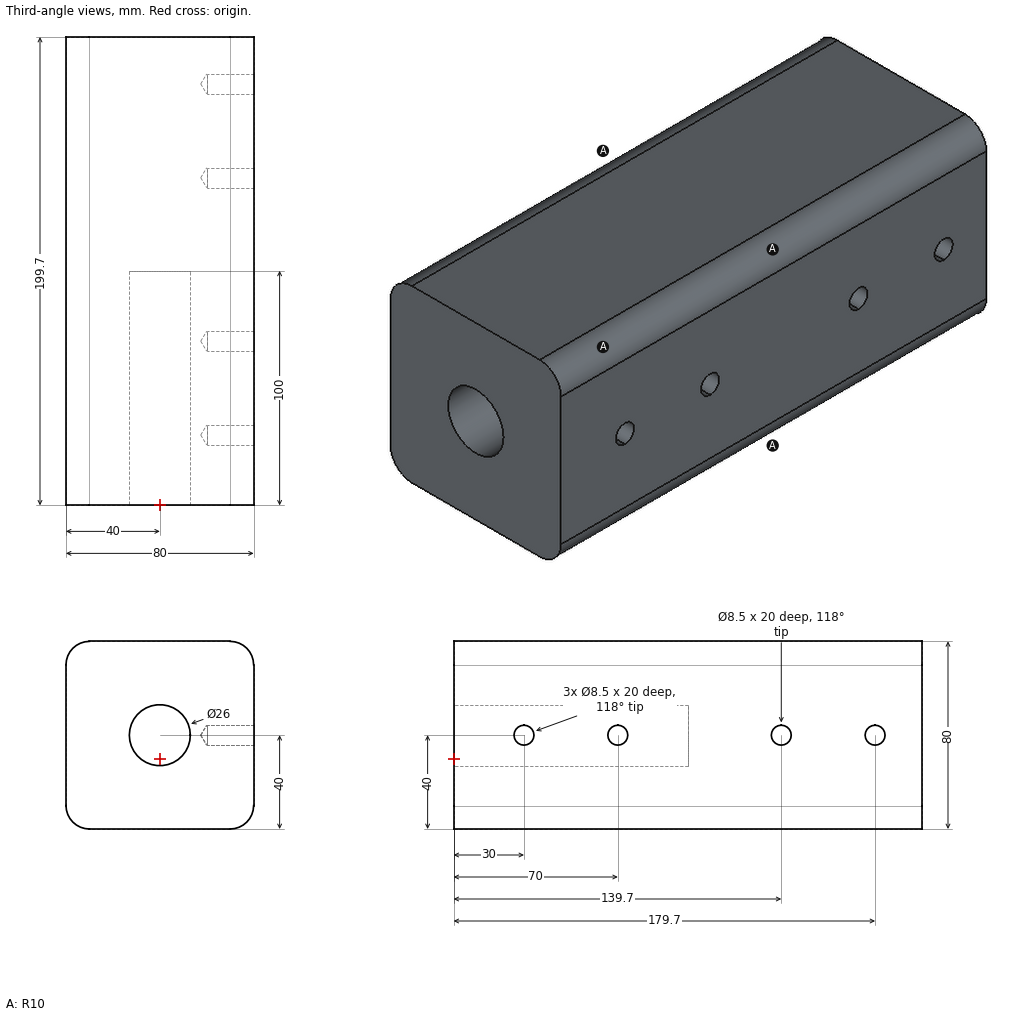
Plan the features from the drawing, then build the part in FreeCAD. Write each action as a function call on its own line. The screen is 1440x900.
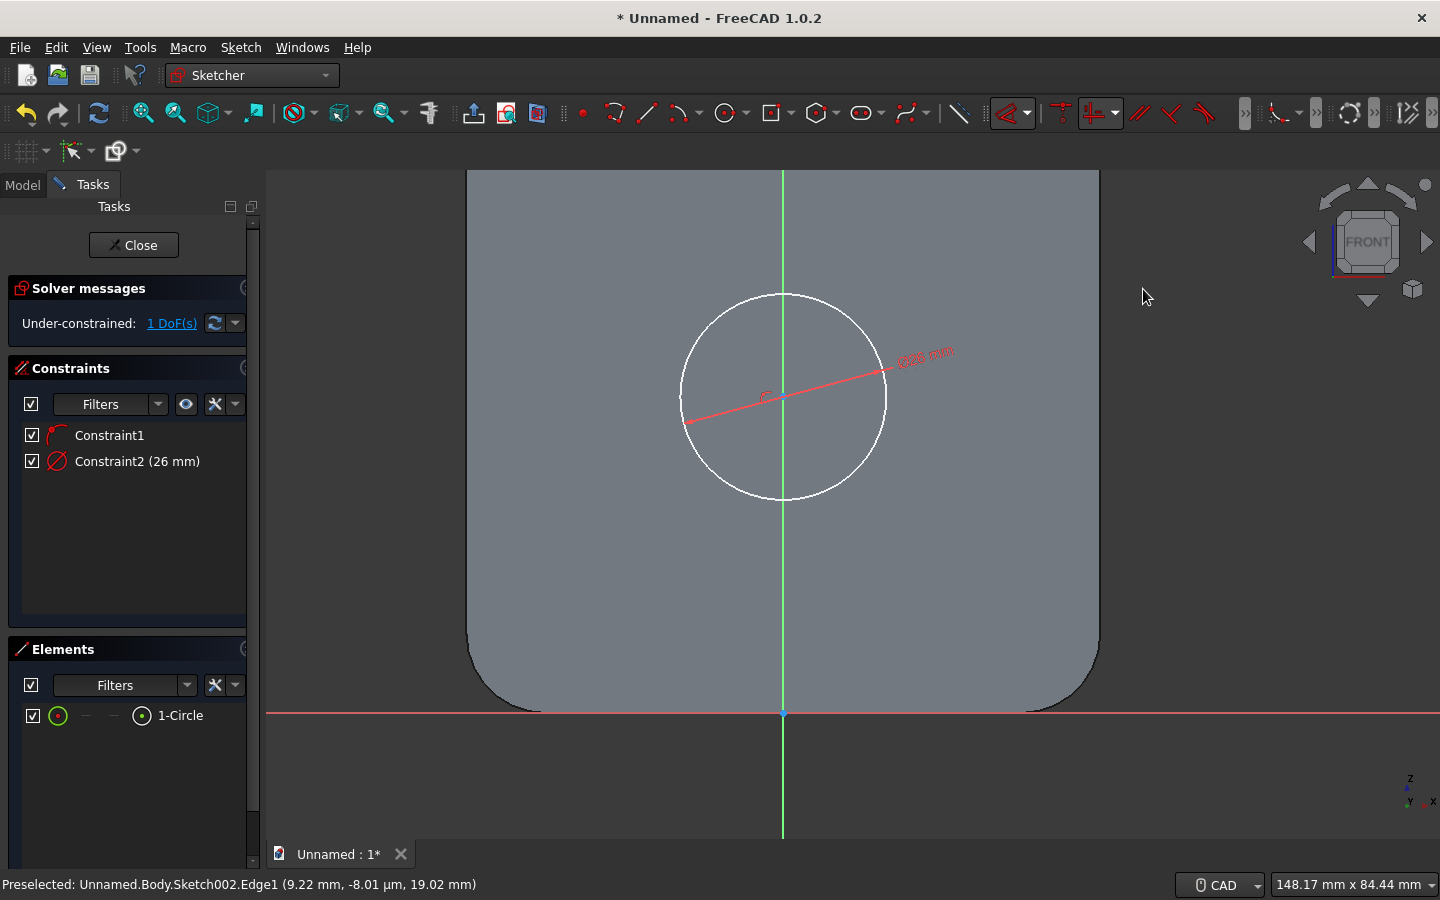
click(783, 397)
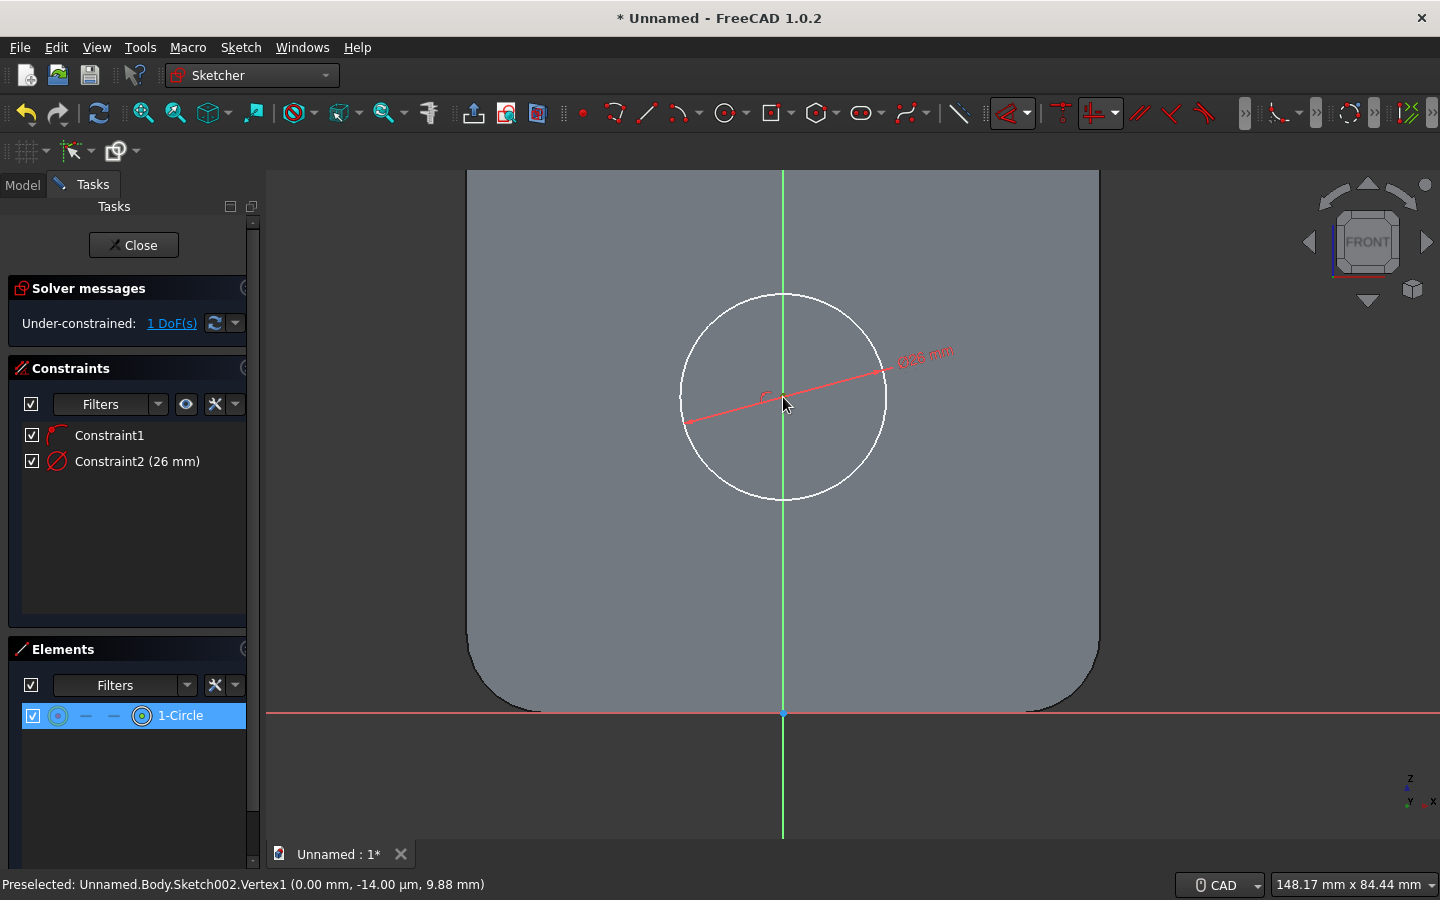
click(1030, 114)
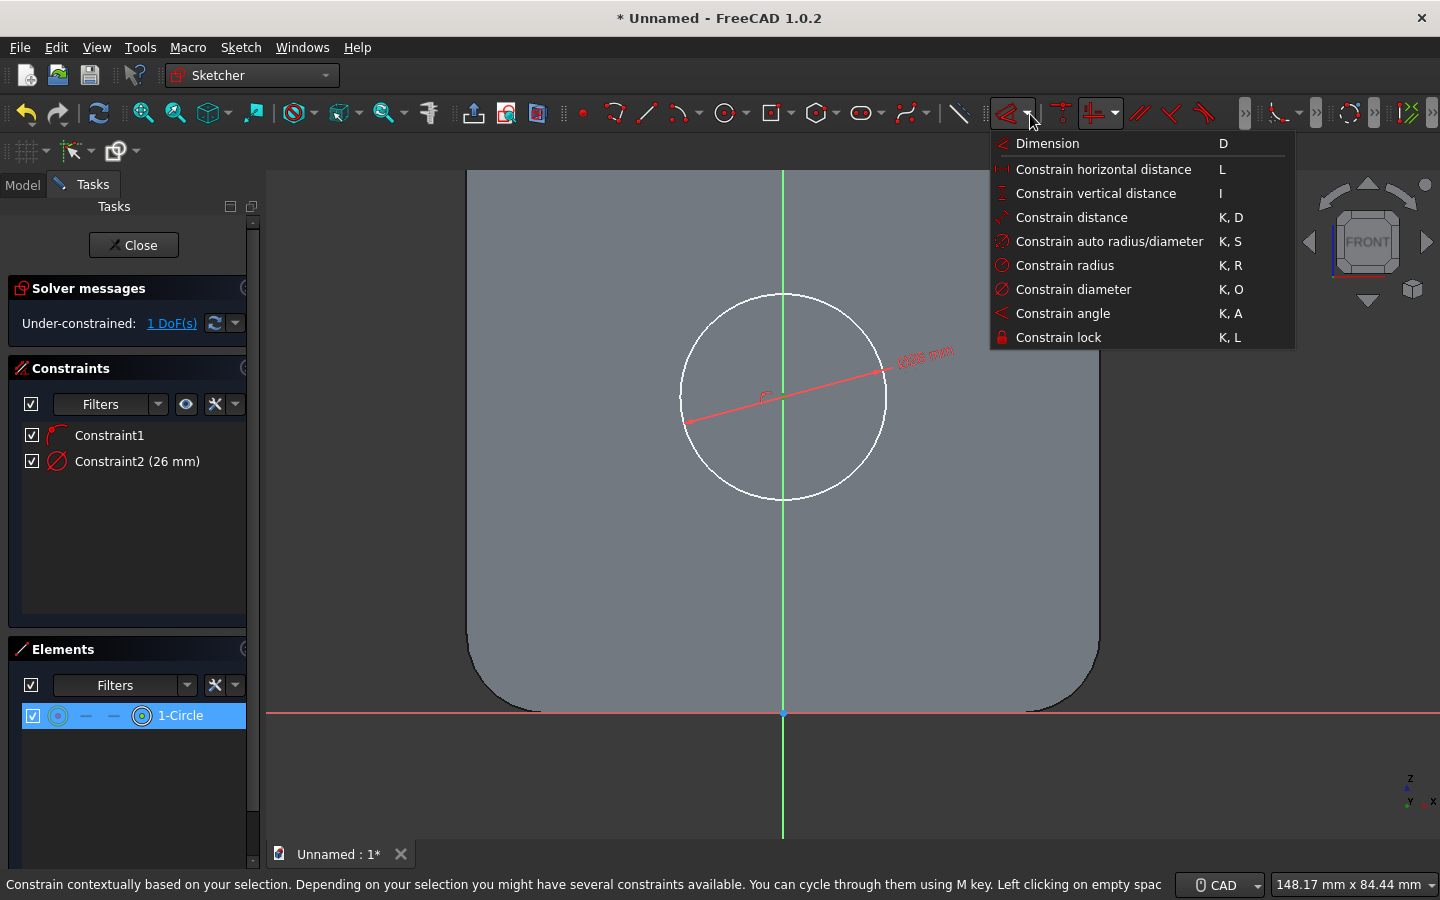
click(1143, 193)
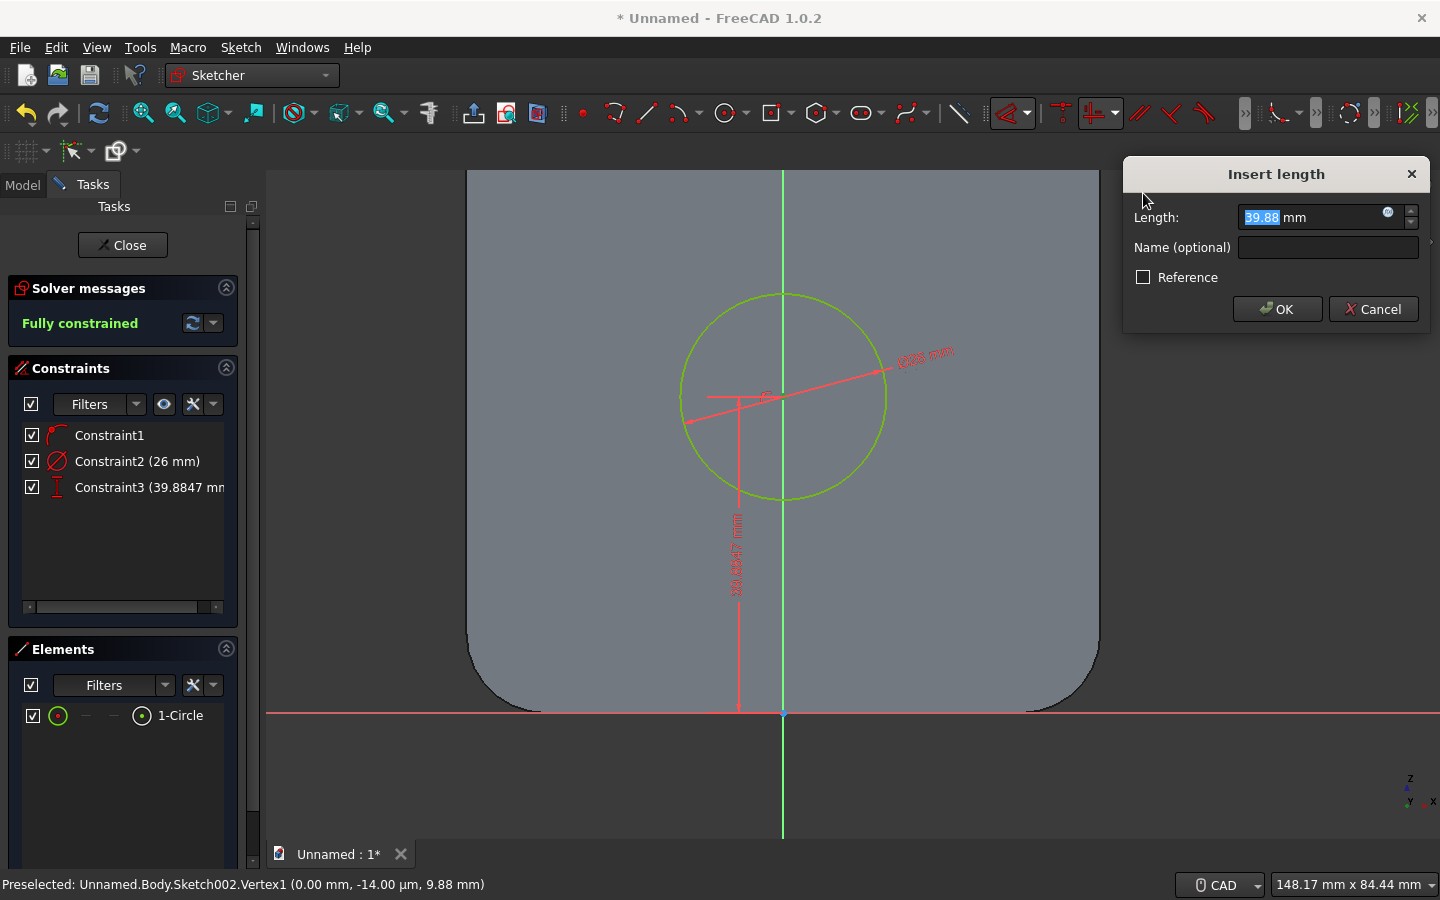
text(40)
key(Return)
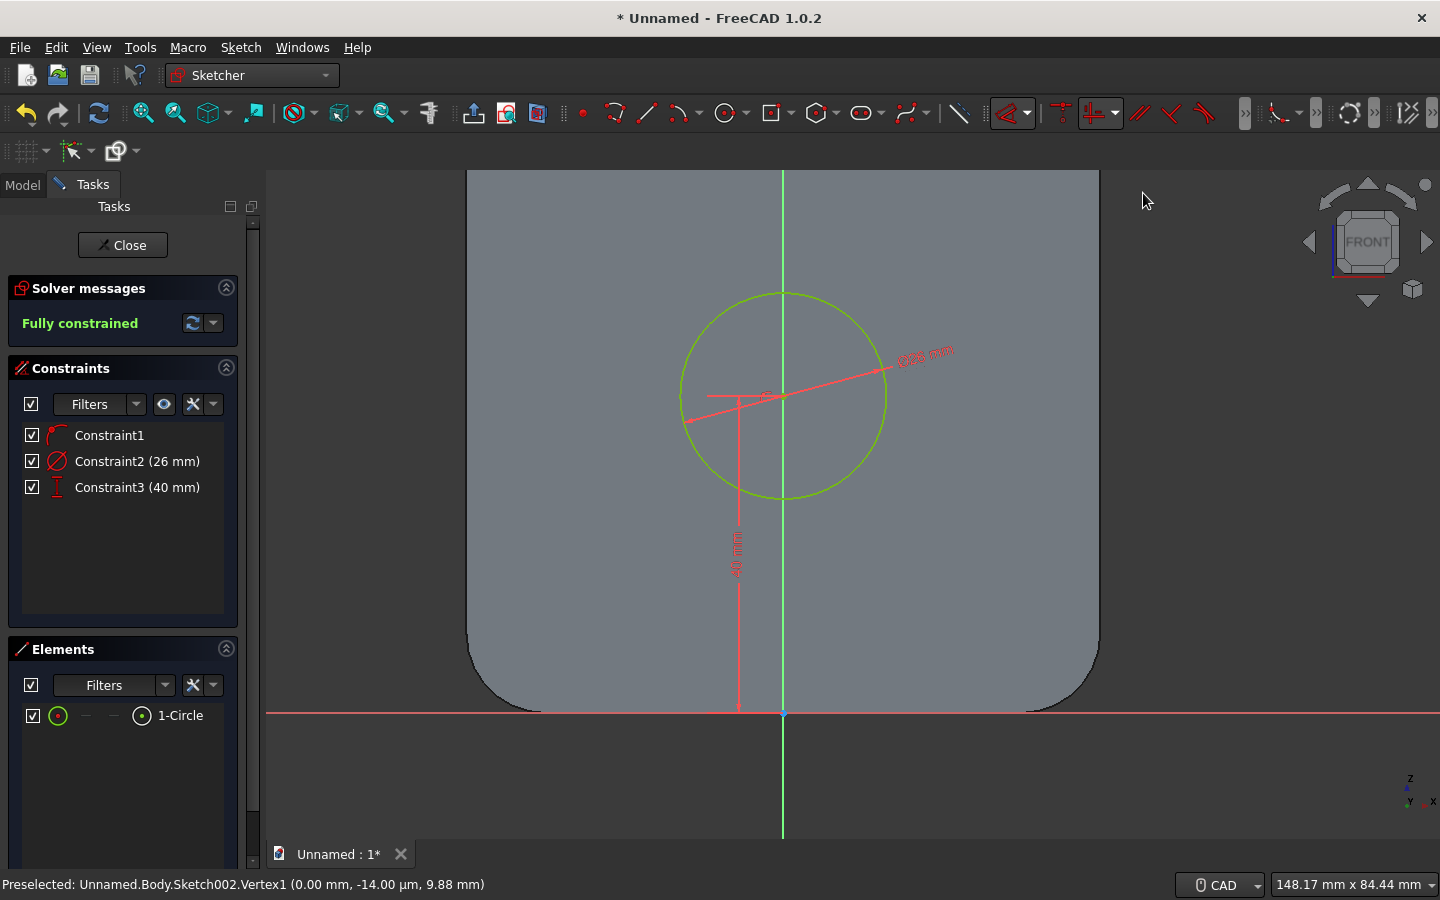
click(123, 245)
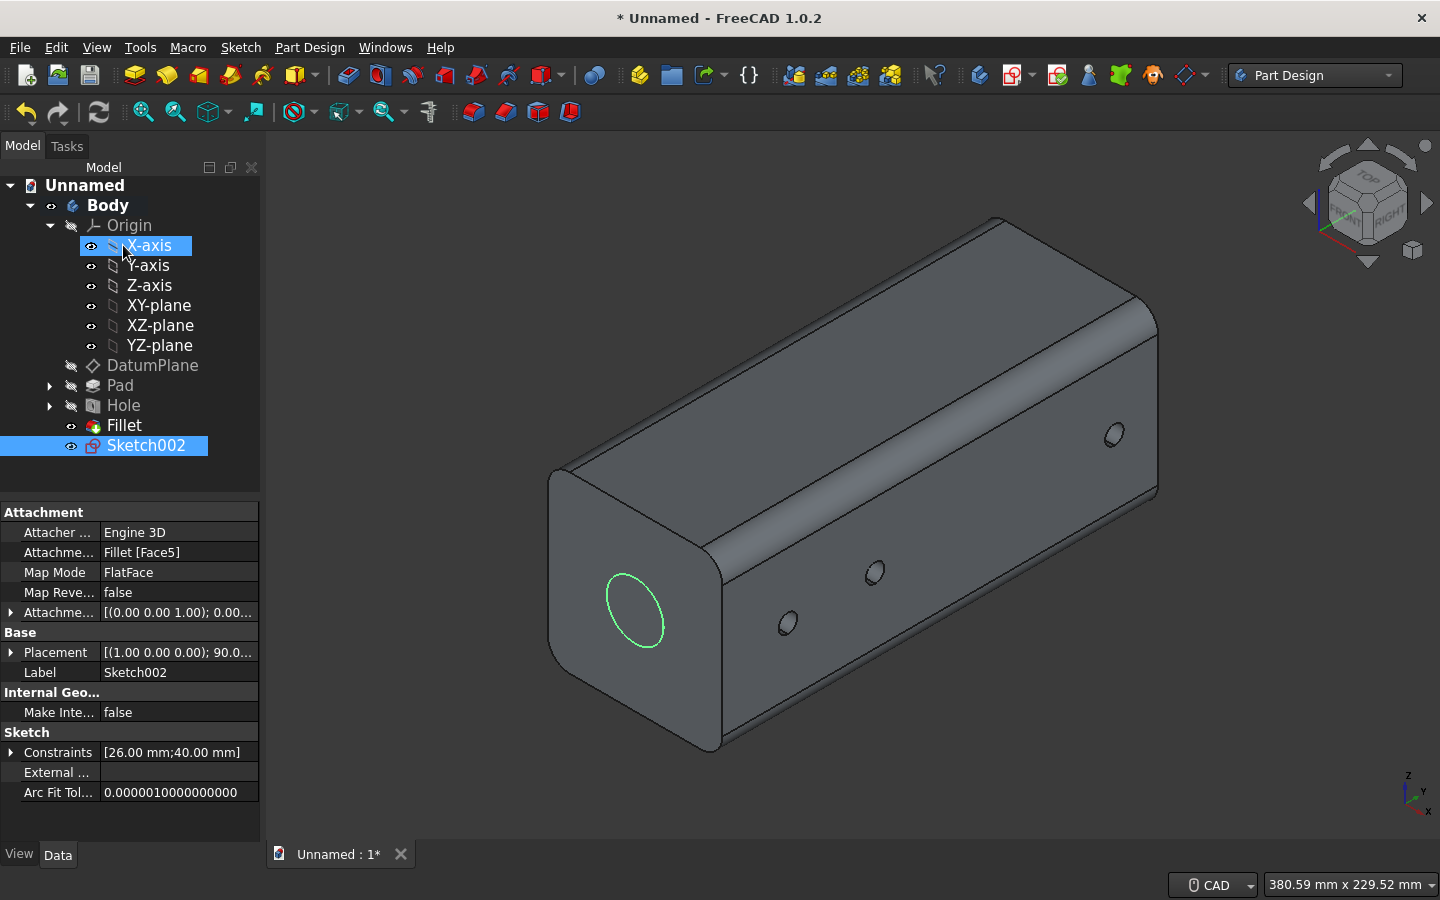
click(350, 76)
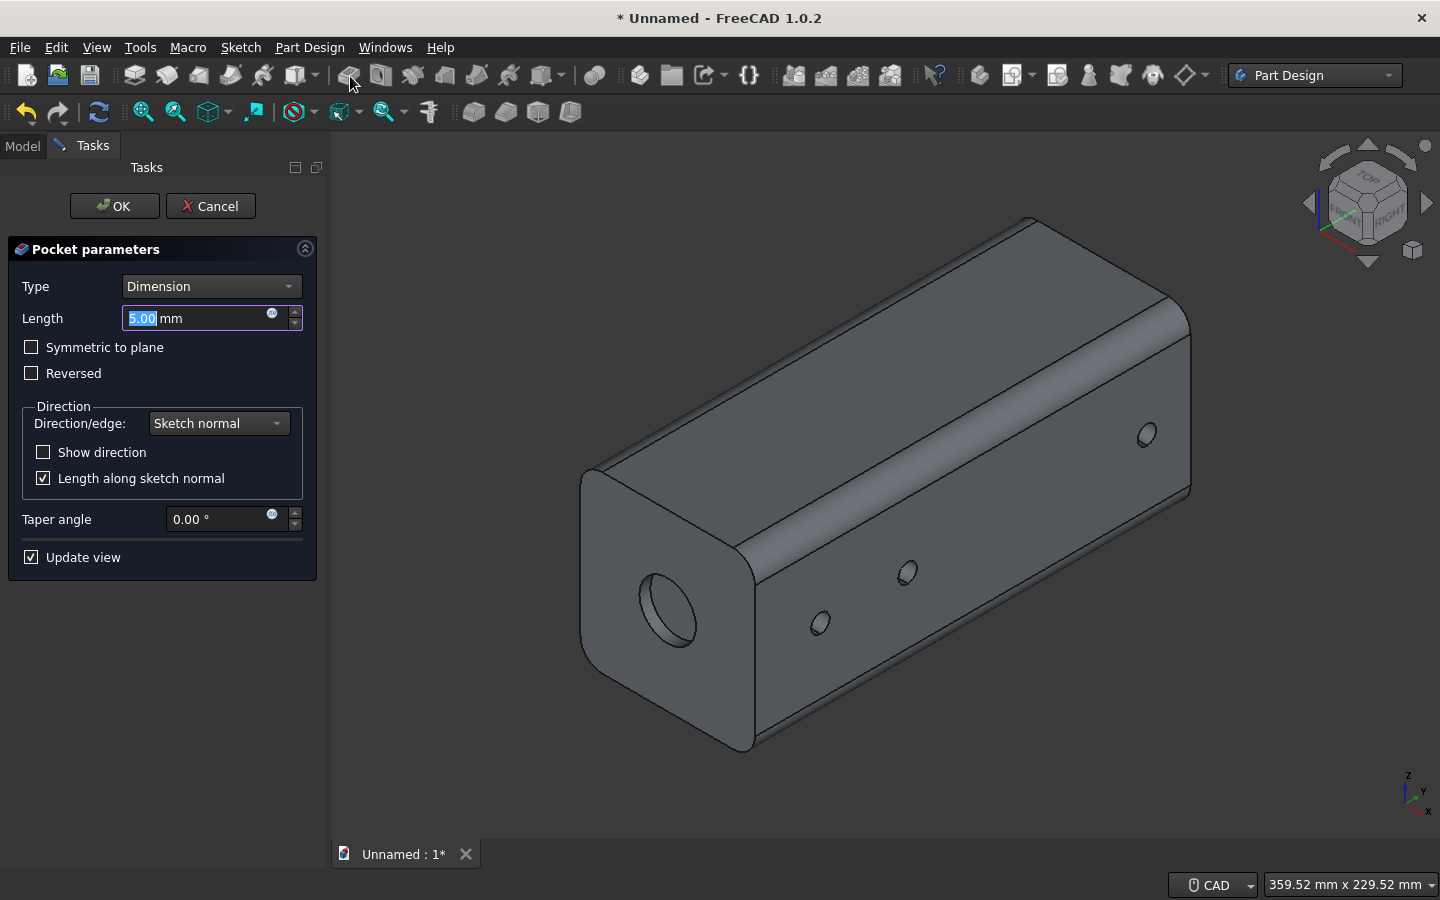
text(100)
key(Tab)